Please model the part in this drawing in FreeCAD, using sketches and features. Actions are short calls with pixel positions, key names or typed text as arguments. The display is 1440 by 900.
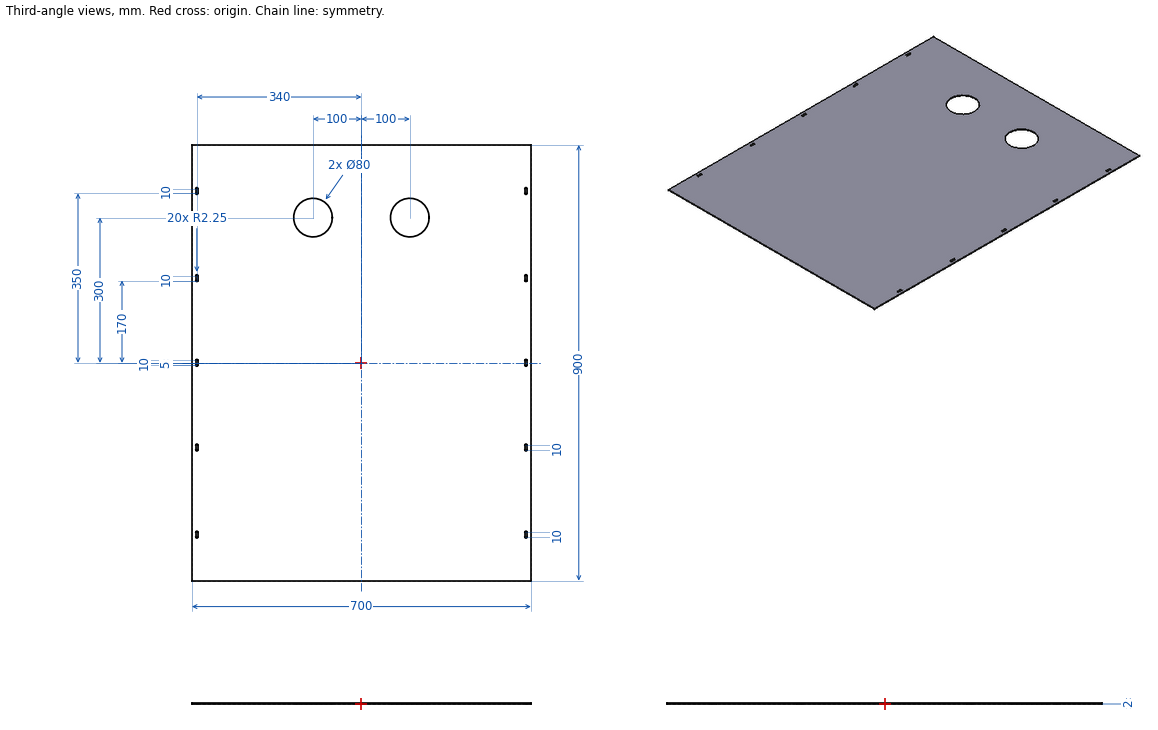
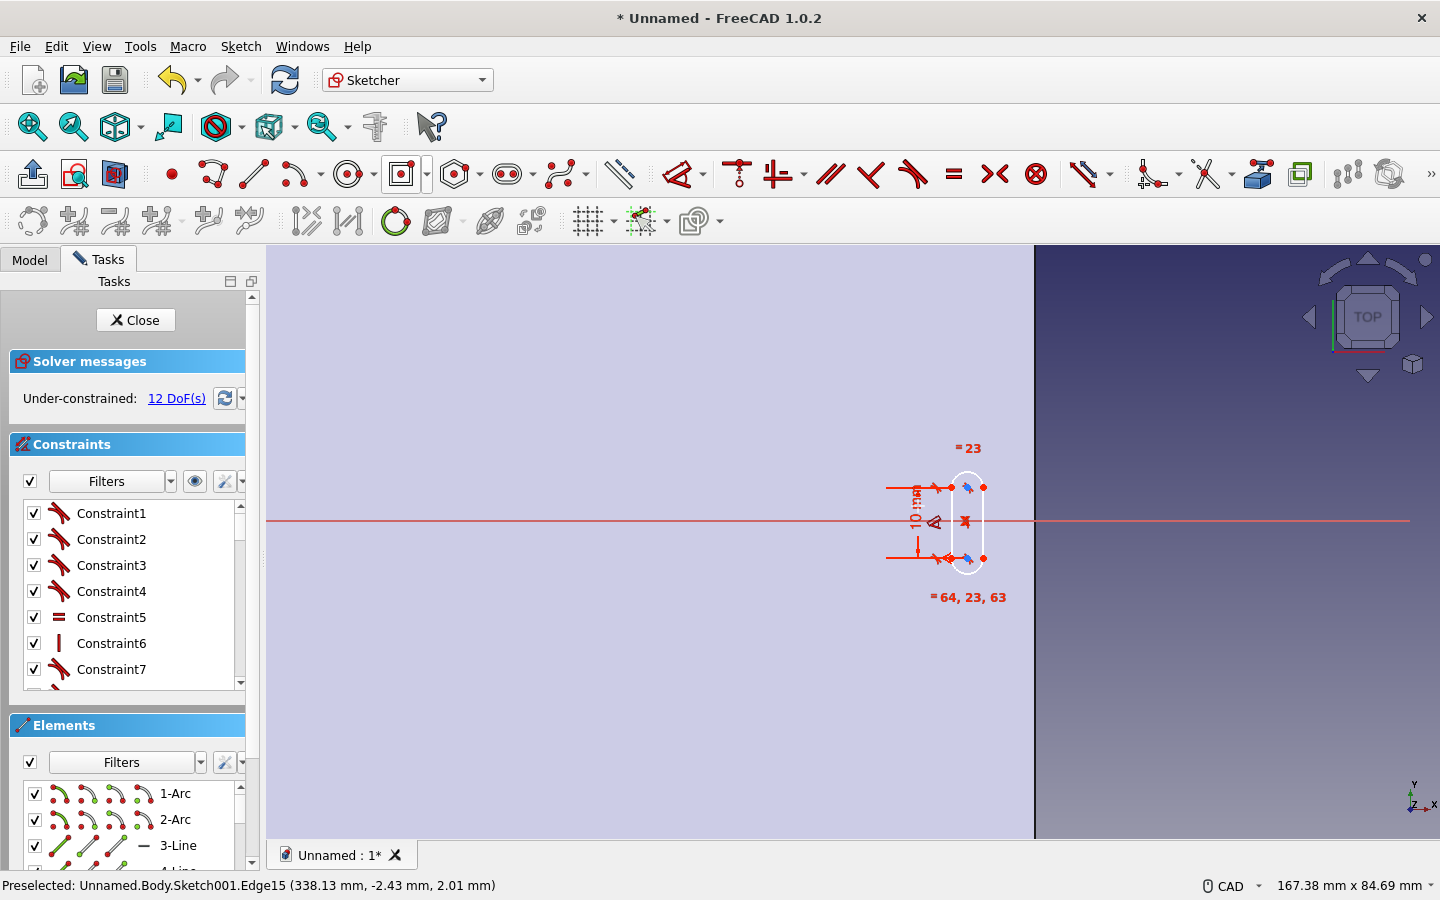
scroll(961, 544, down, 13)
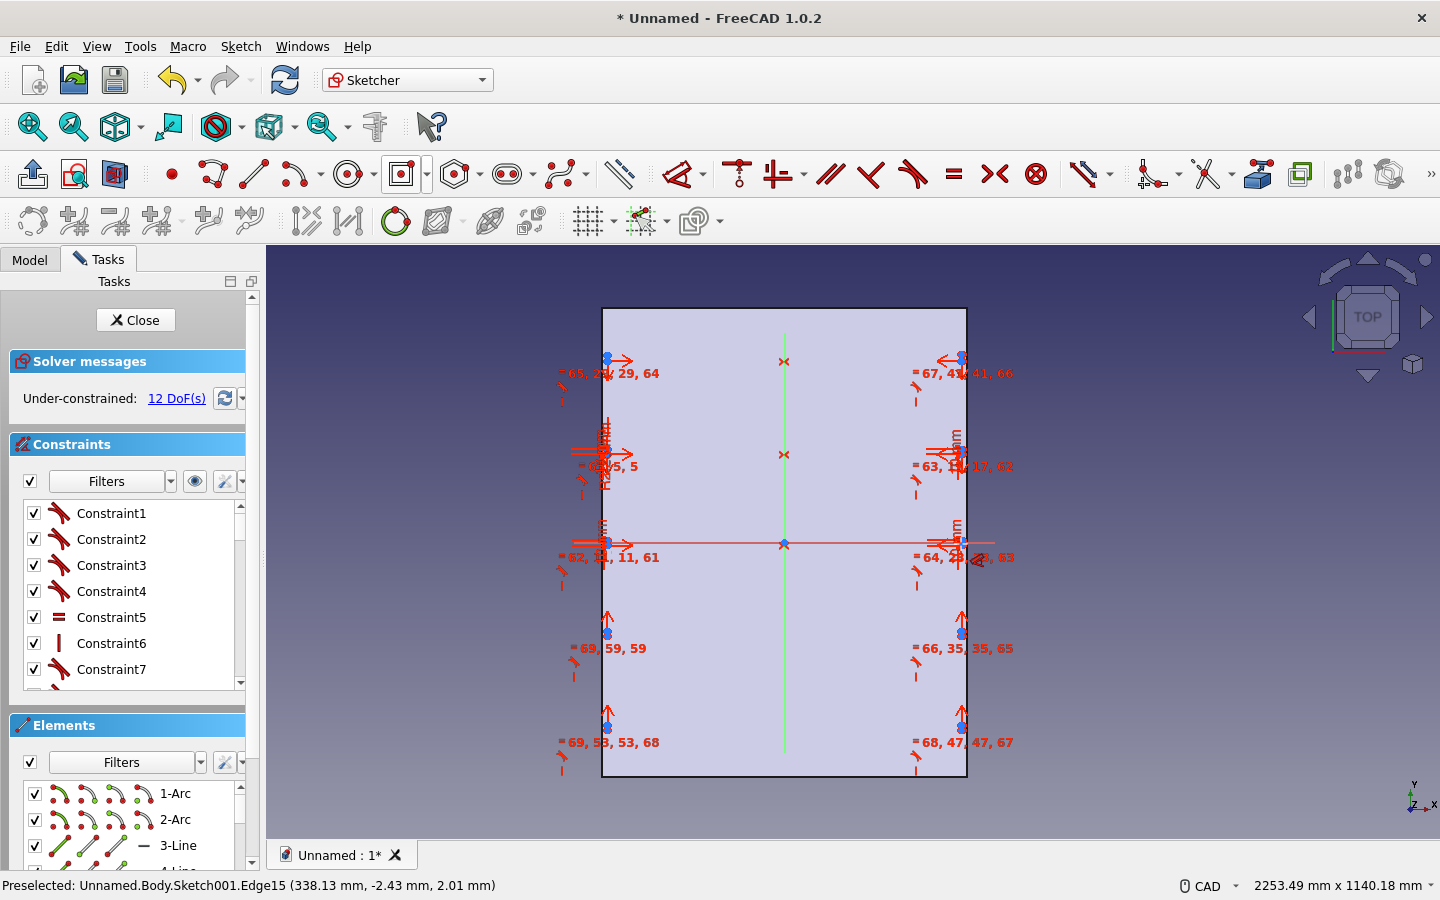
scroll(606, 359, up, 11)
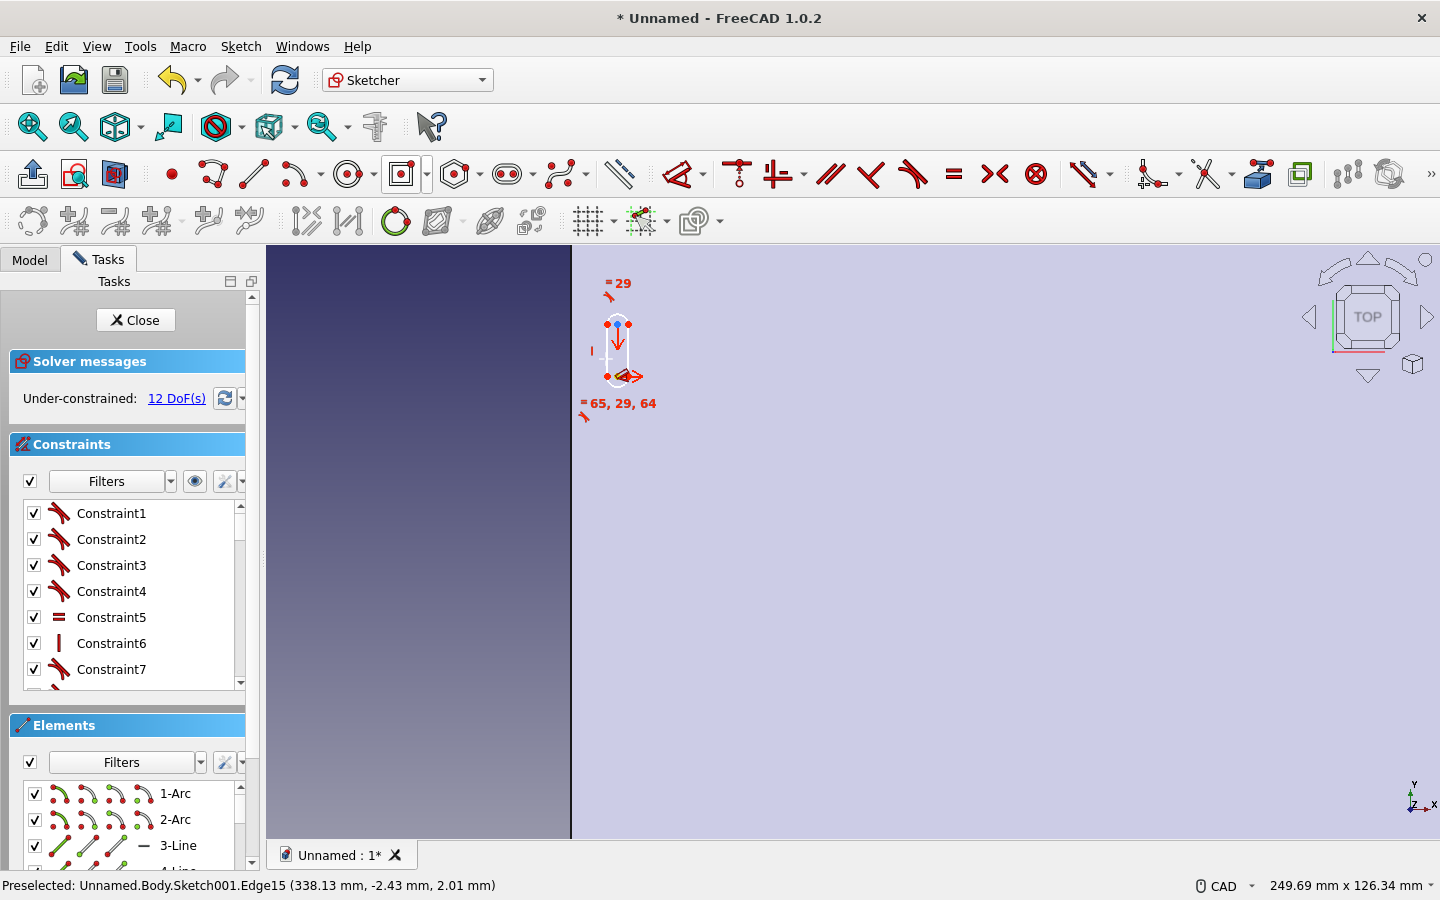
click(607, 361)
click(573, 351)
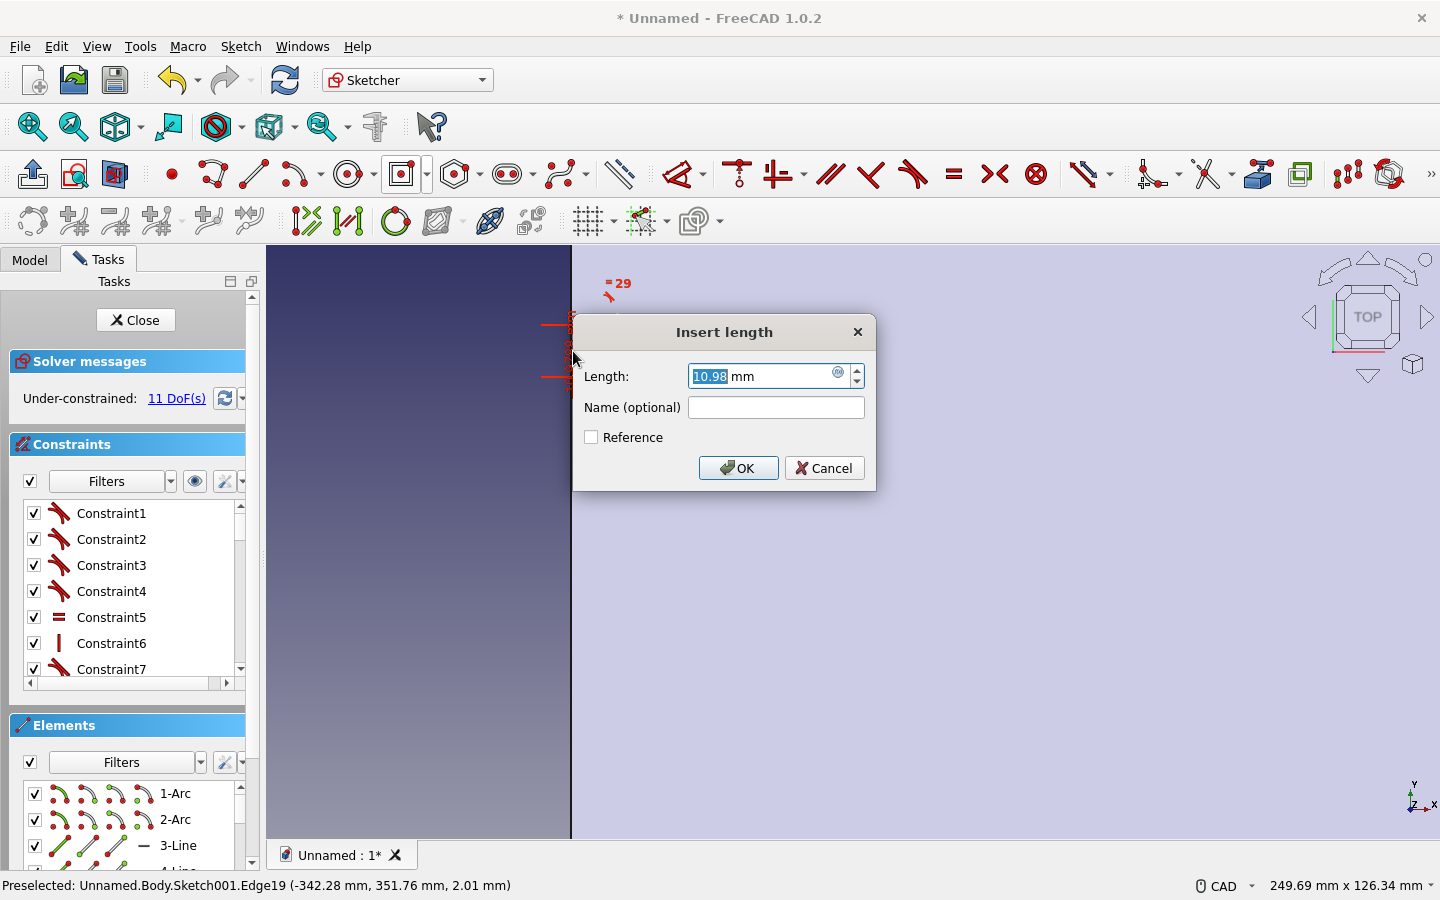
text(10)
key(Return)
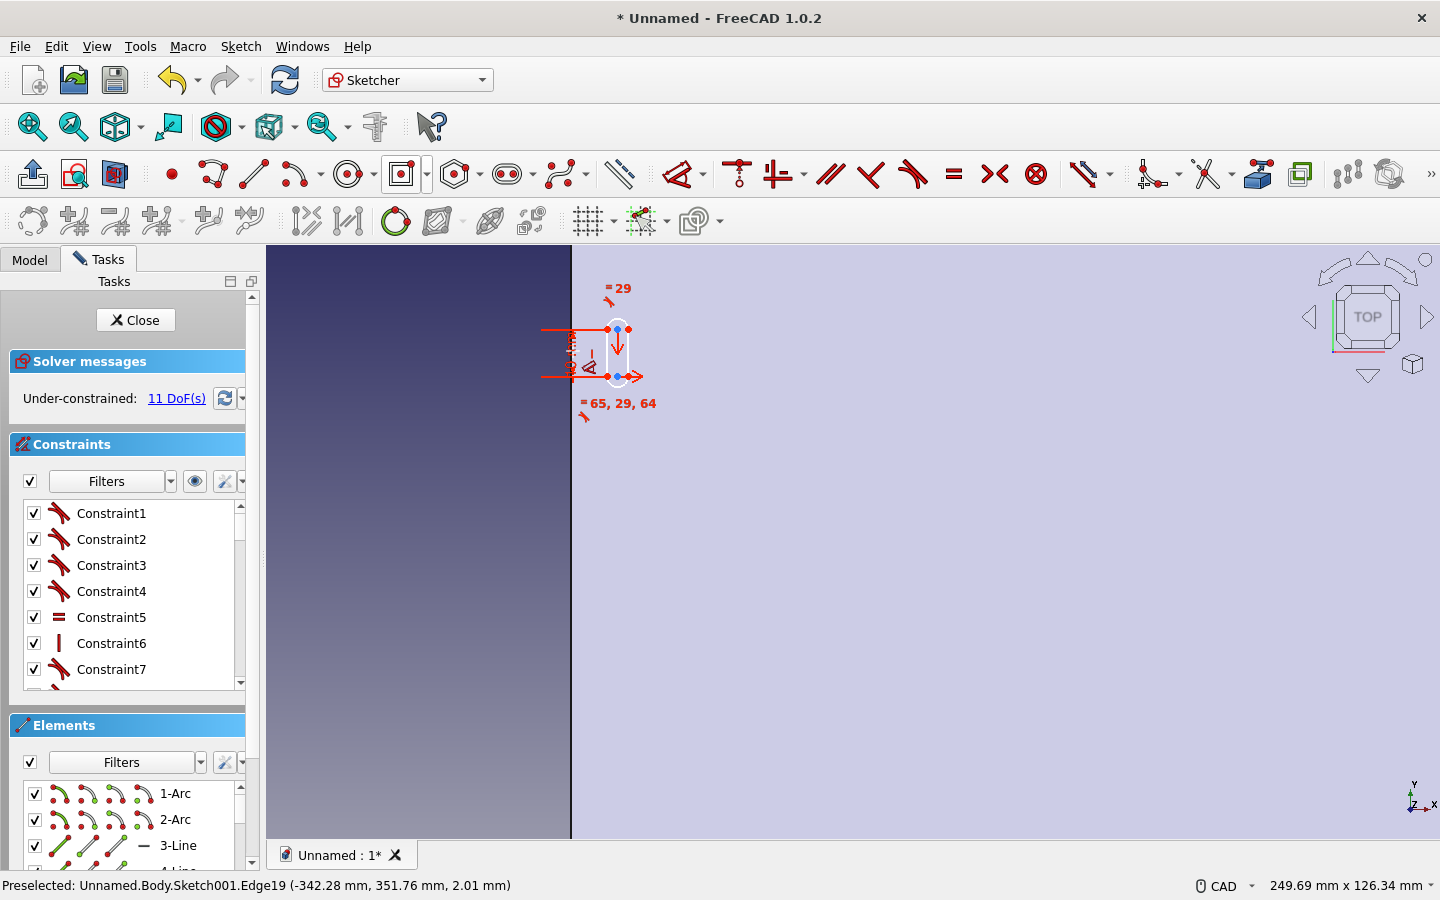
scroll(606, 358, down, 11)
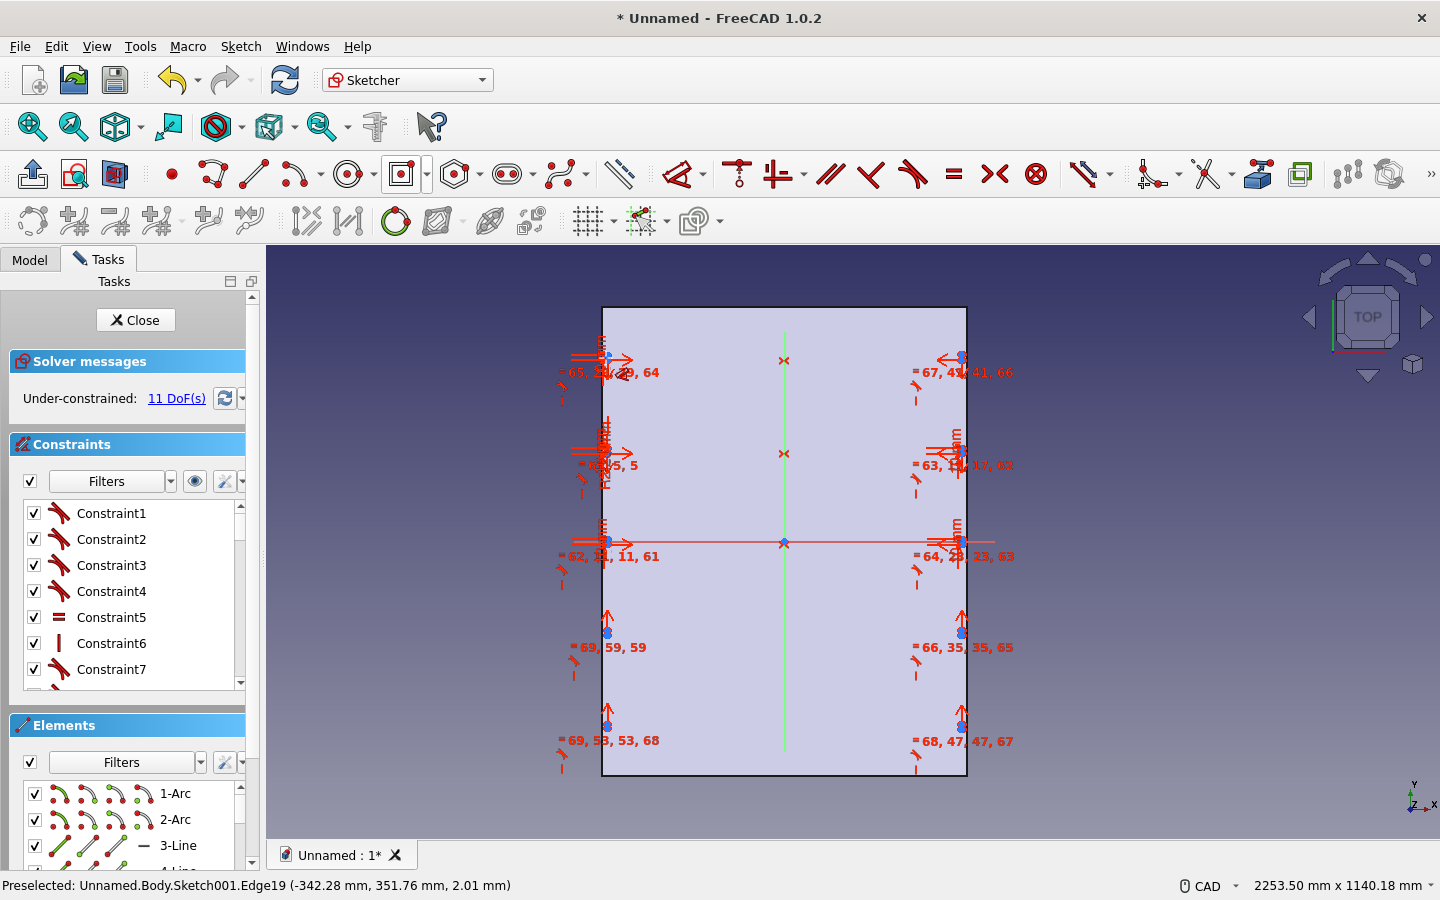
scroll(961, 634, up, 12)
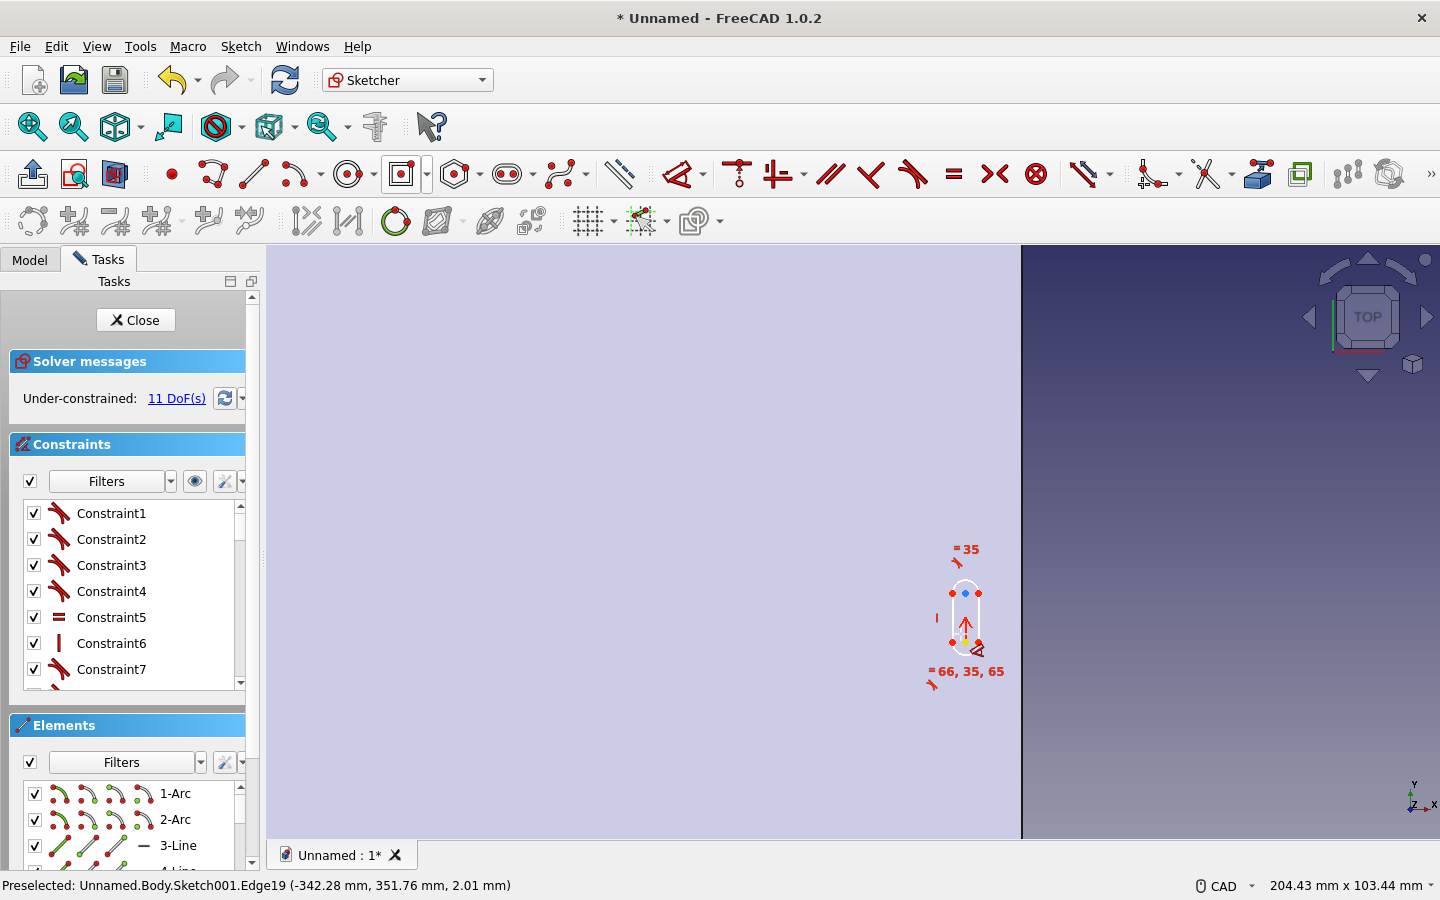
click(953, 628)
click(919, 618)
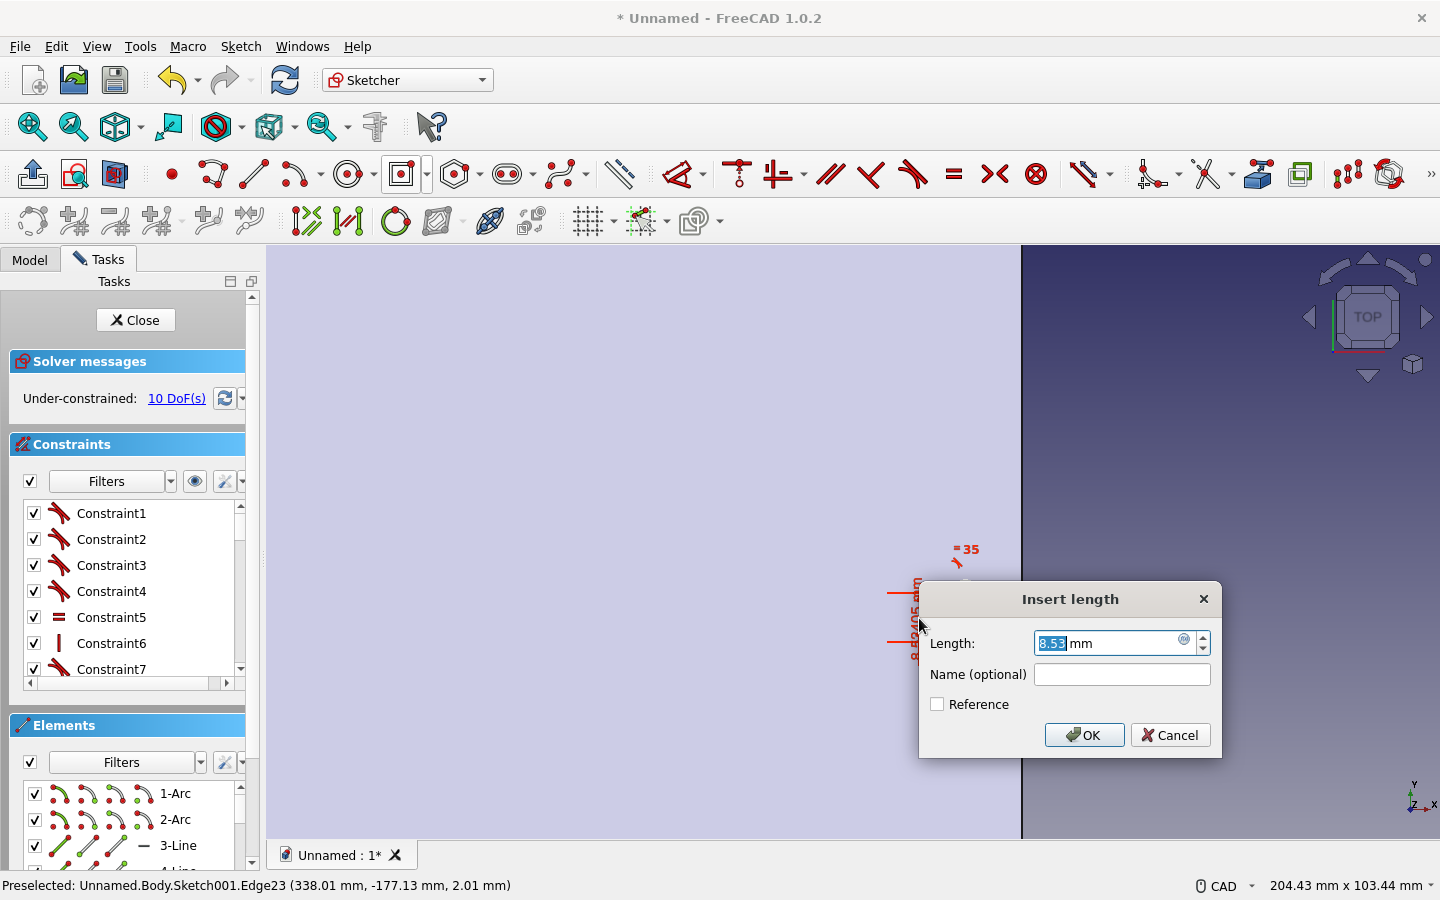
text(10)
key(Return)